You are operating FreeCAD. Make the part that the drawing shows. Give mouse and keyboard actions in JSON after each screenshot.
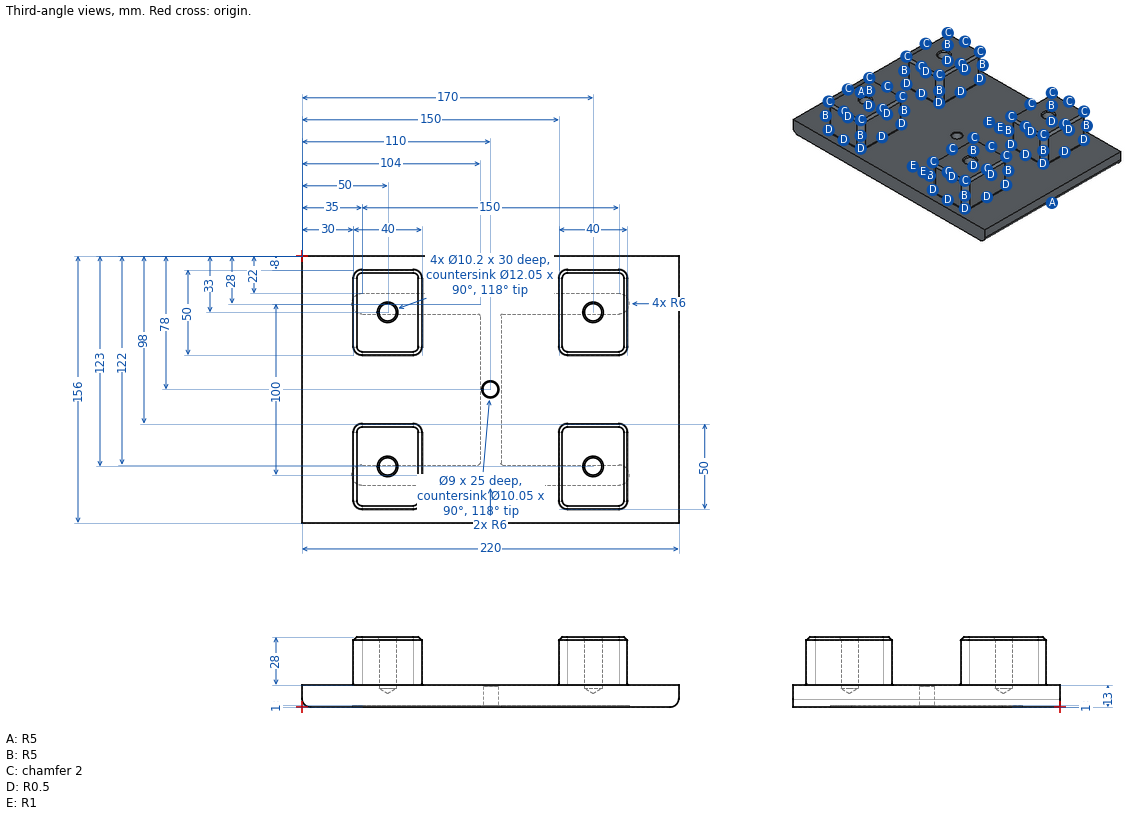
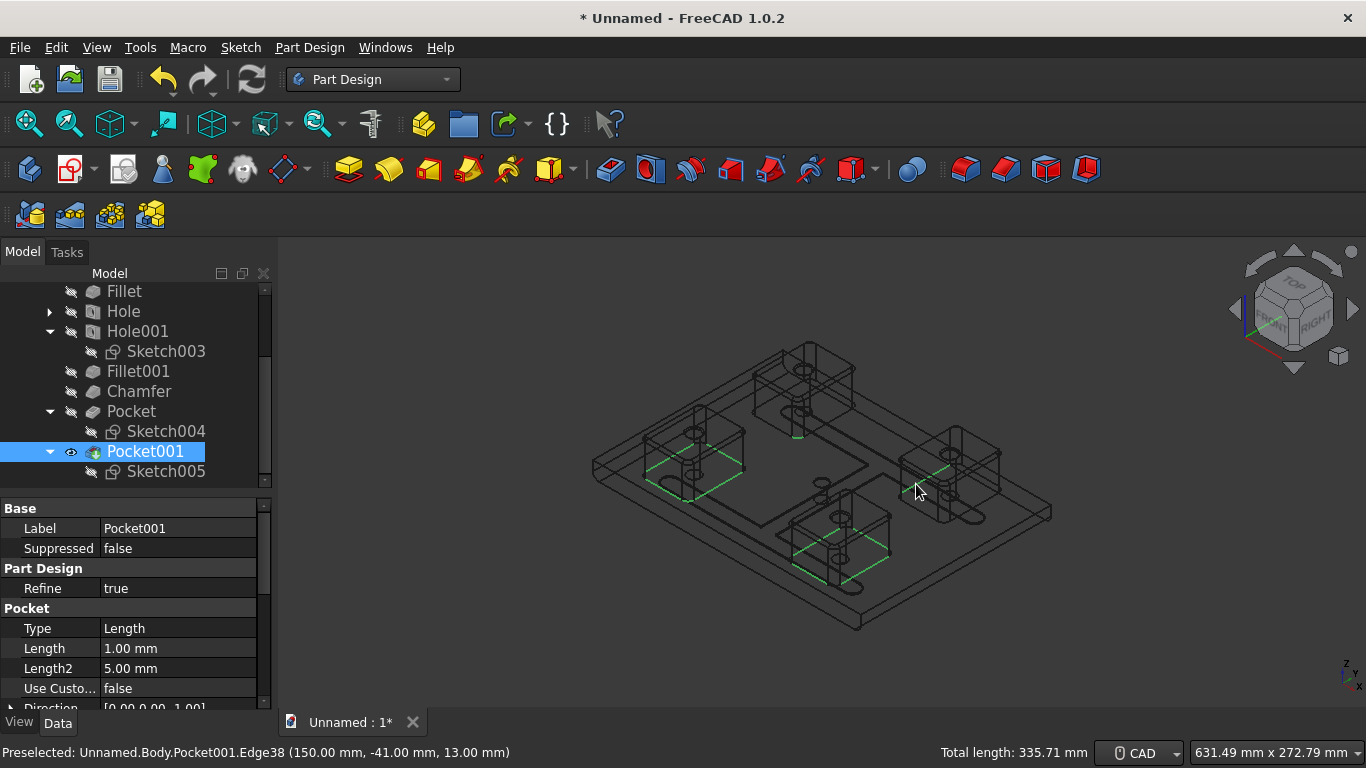
{"action": "left_click", "coordinate": [980, 475], "text": "ctrl"}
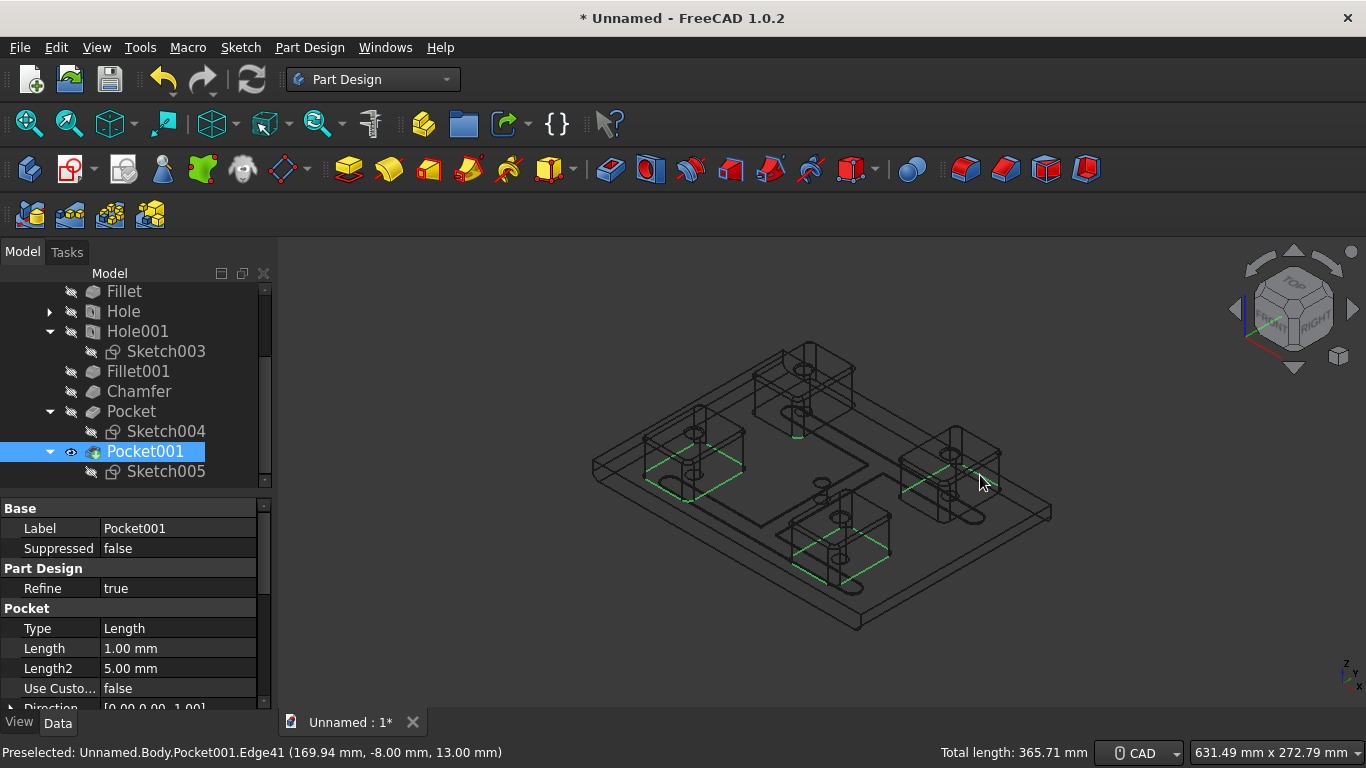
{"action": "left_click", "coordinate": [974, 506], "text": "ctrl"}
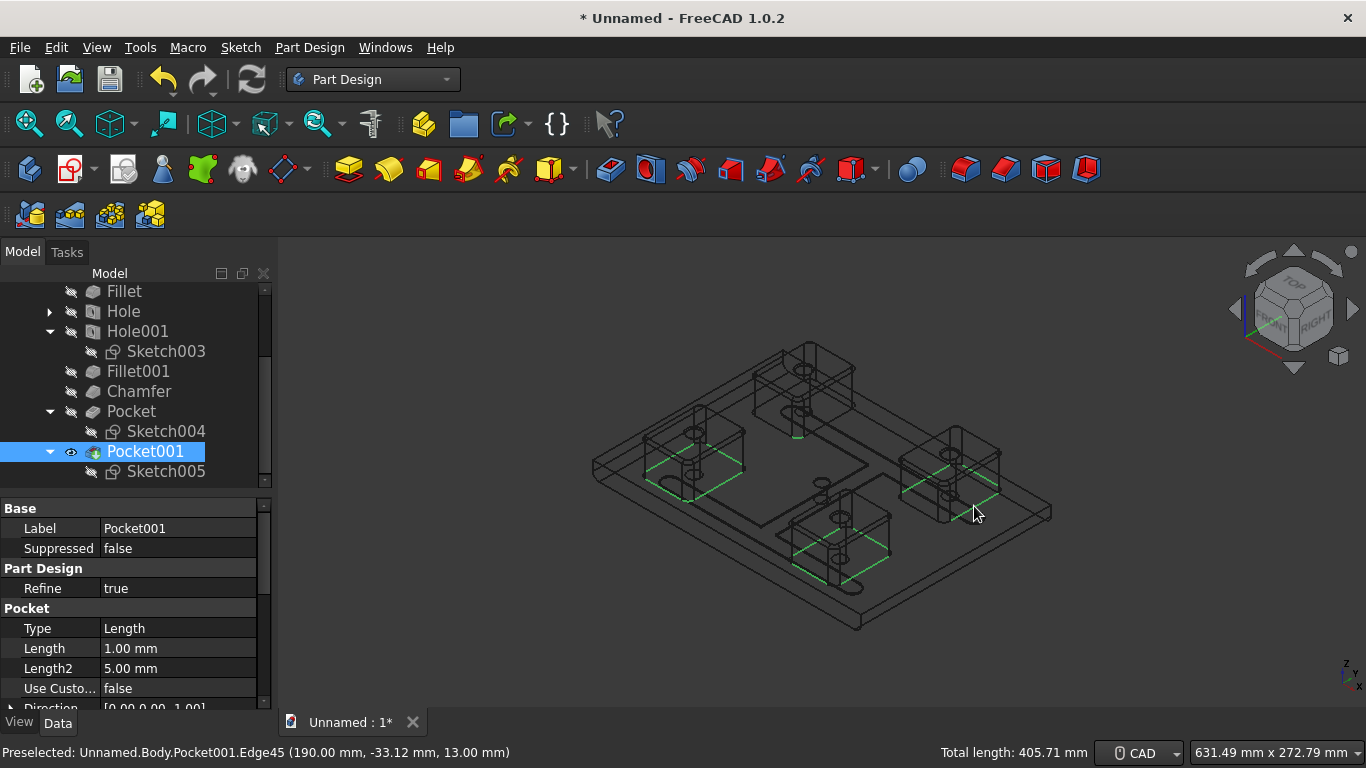
{"action": "left_click", "coordinate": [919, 510], "text": "ctrl"}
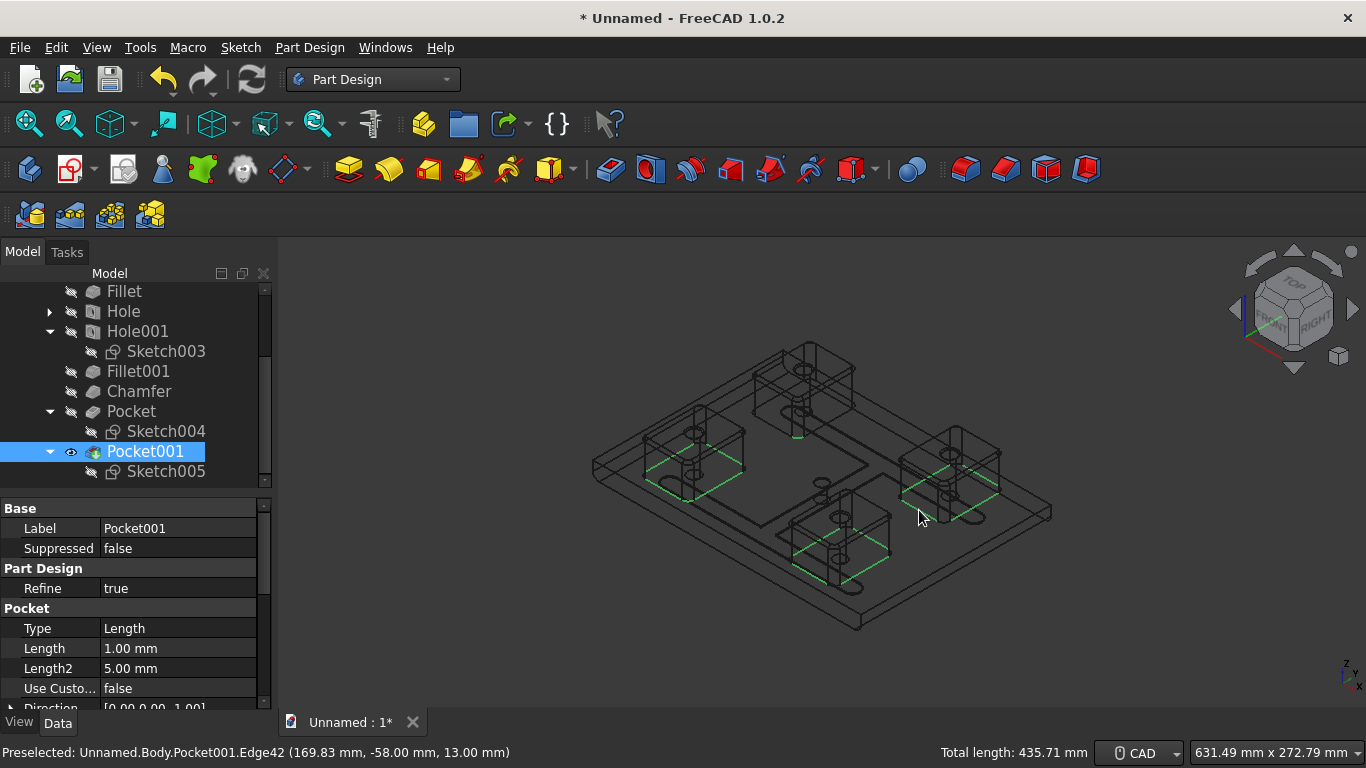
{"action": "left_click", "coordinate": [828, 422], "text": "ctrl"}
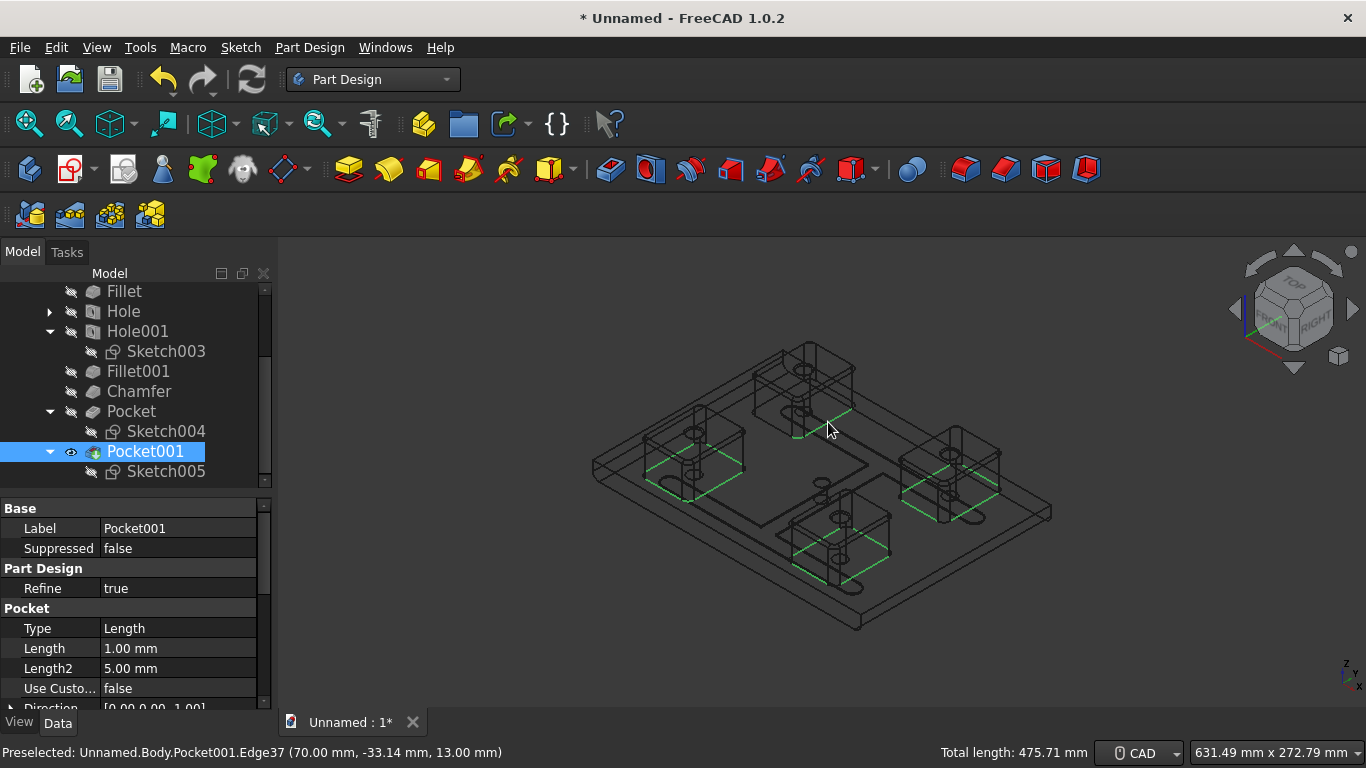
{"action": "left_click", "coordinate": [773, 425], "text": "ctrl"}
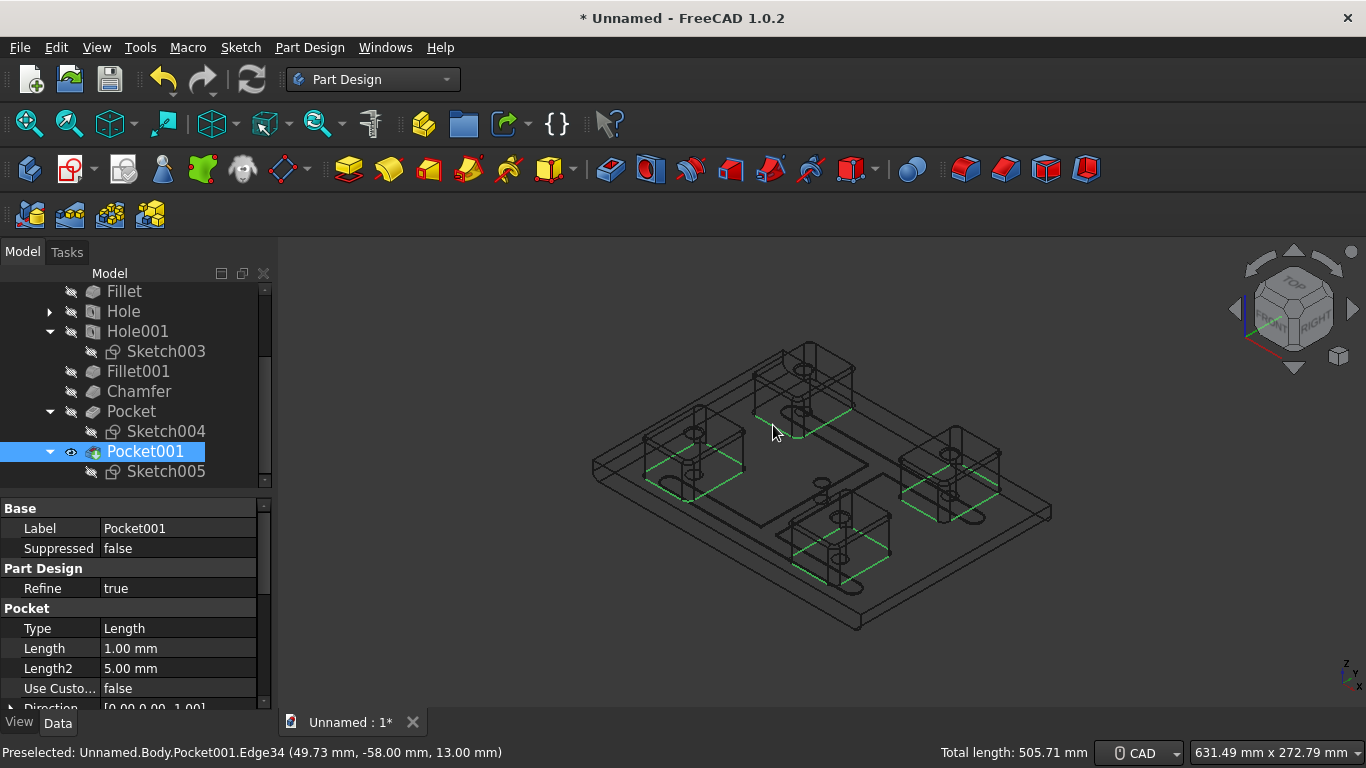
{"action": "left_click", "coordinate": [770, 399], "text": "ctrl"}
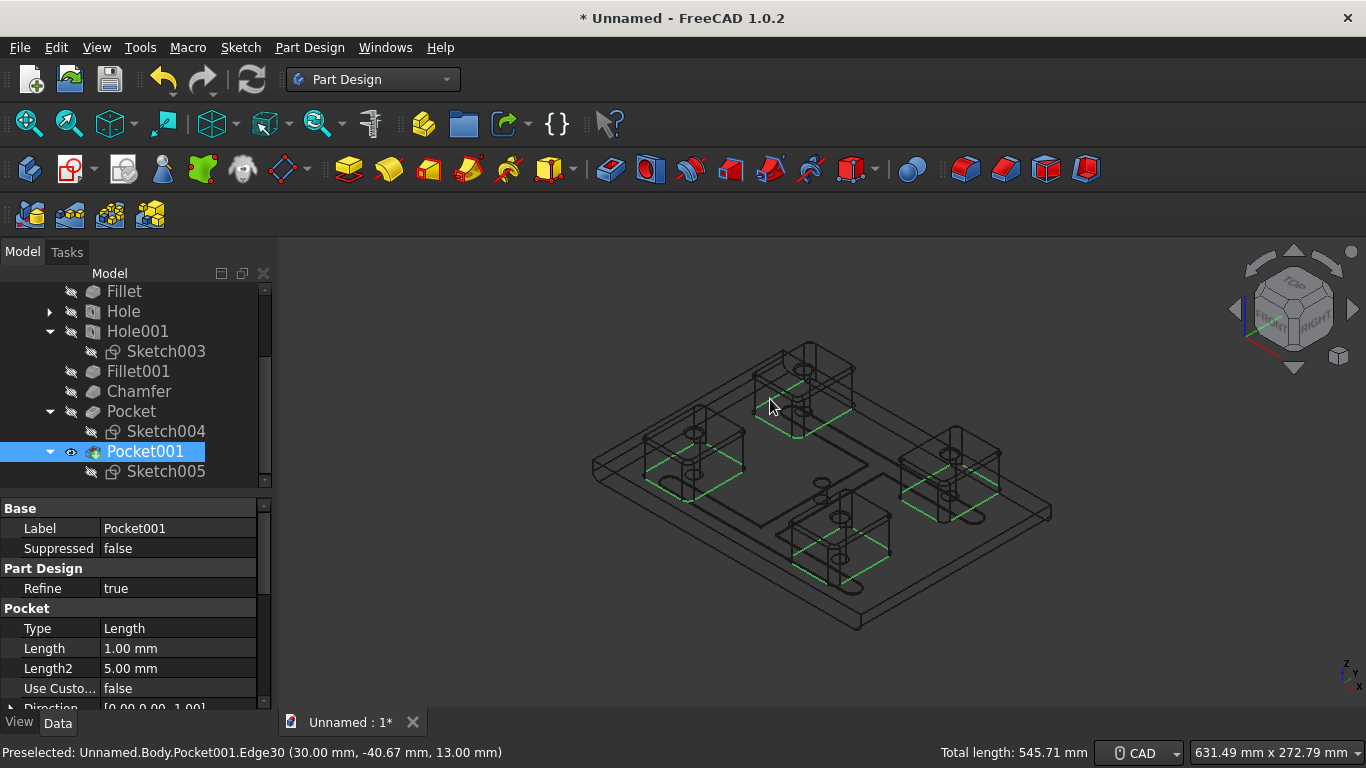
{"action": "left_click", "coordinate": [834, 390], "text": "ctrl"}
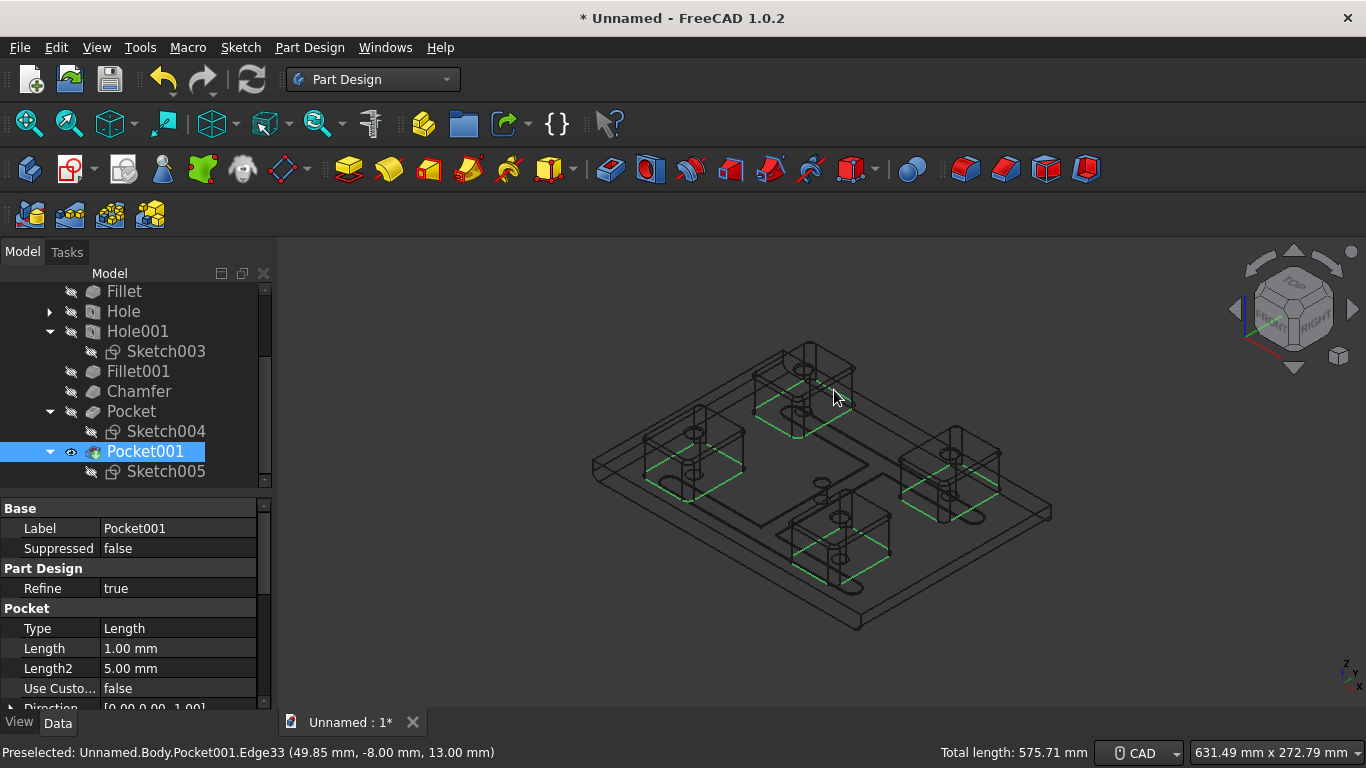
{"action": "left_click", "coordinate": [834, 585], "text": "ctrl"}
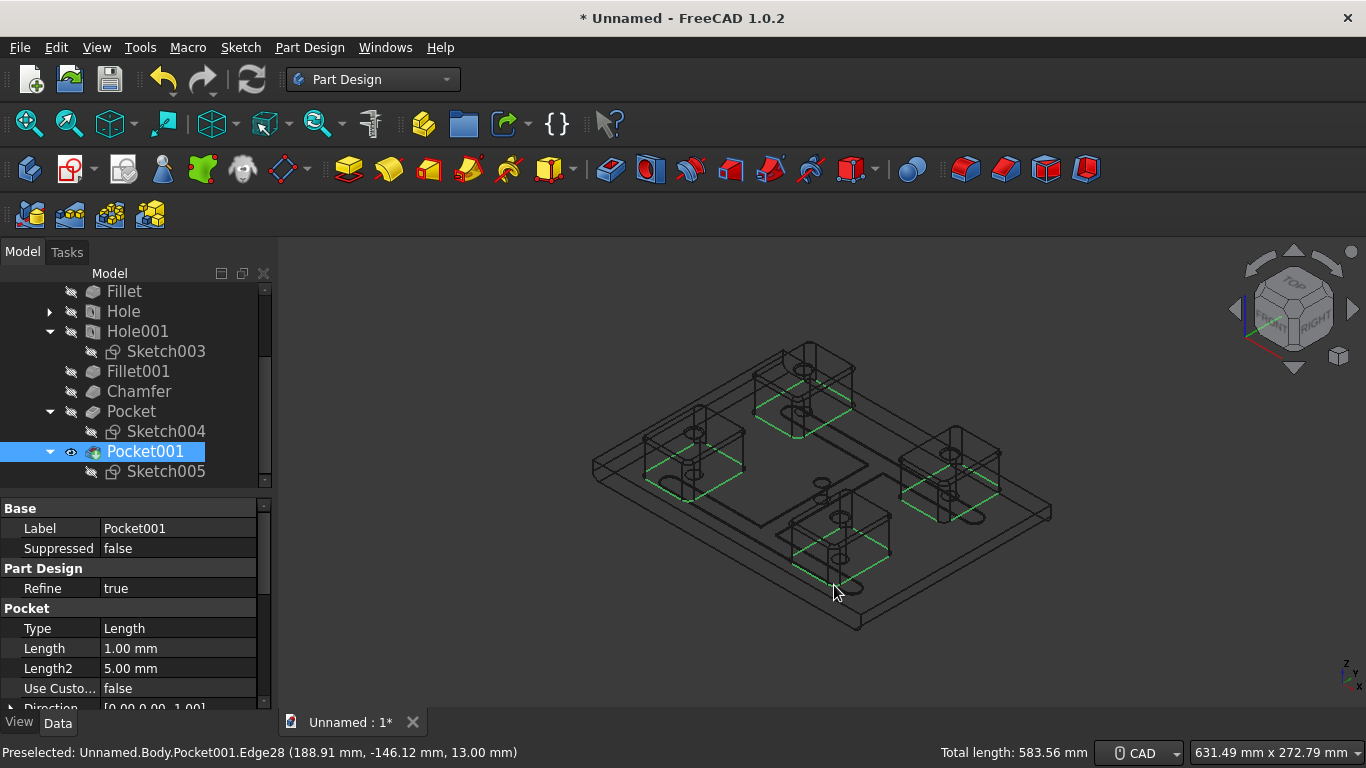
{"action": "left_click", "coordinate": [944, 522], "text": "ctrl"}